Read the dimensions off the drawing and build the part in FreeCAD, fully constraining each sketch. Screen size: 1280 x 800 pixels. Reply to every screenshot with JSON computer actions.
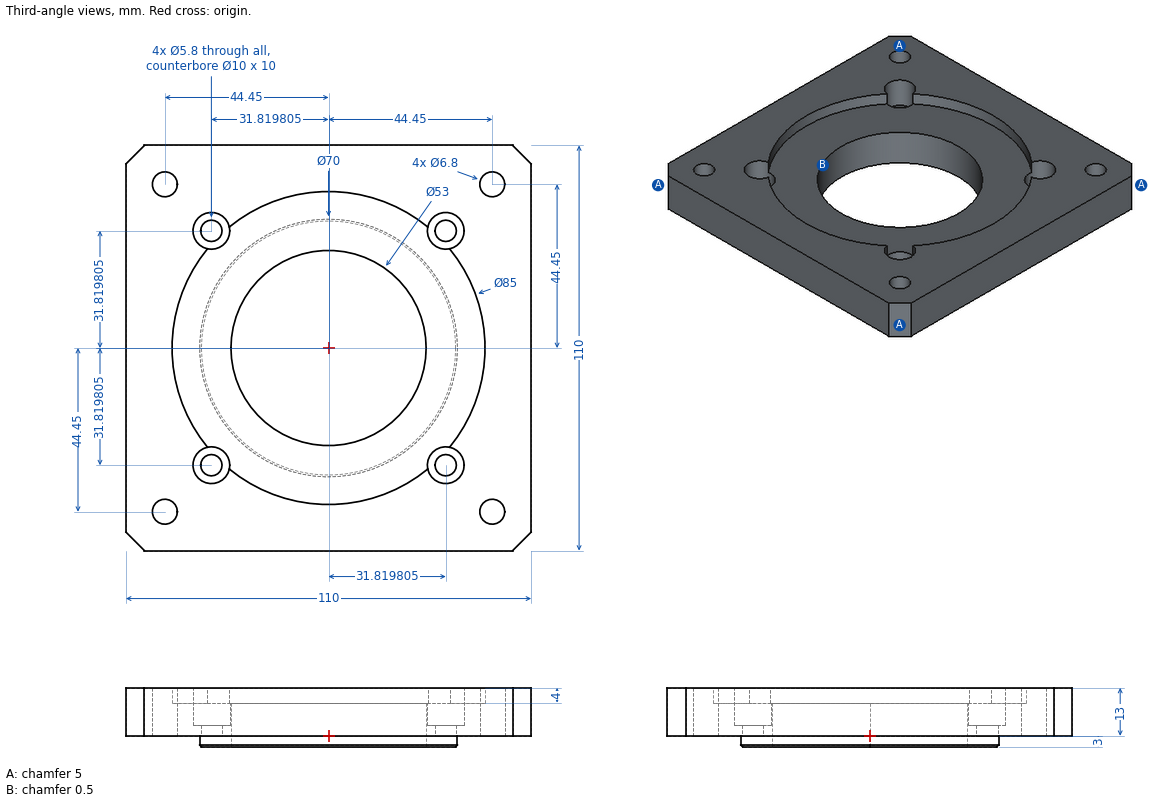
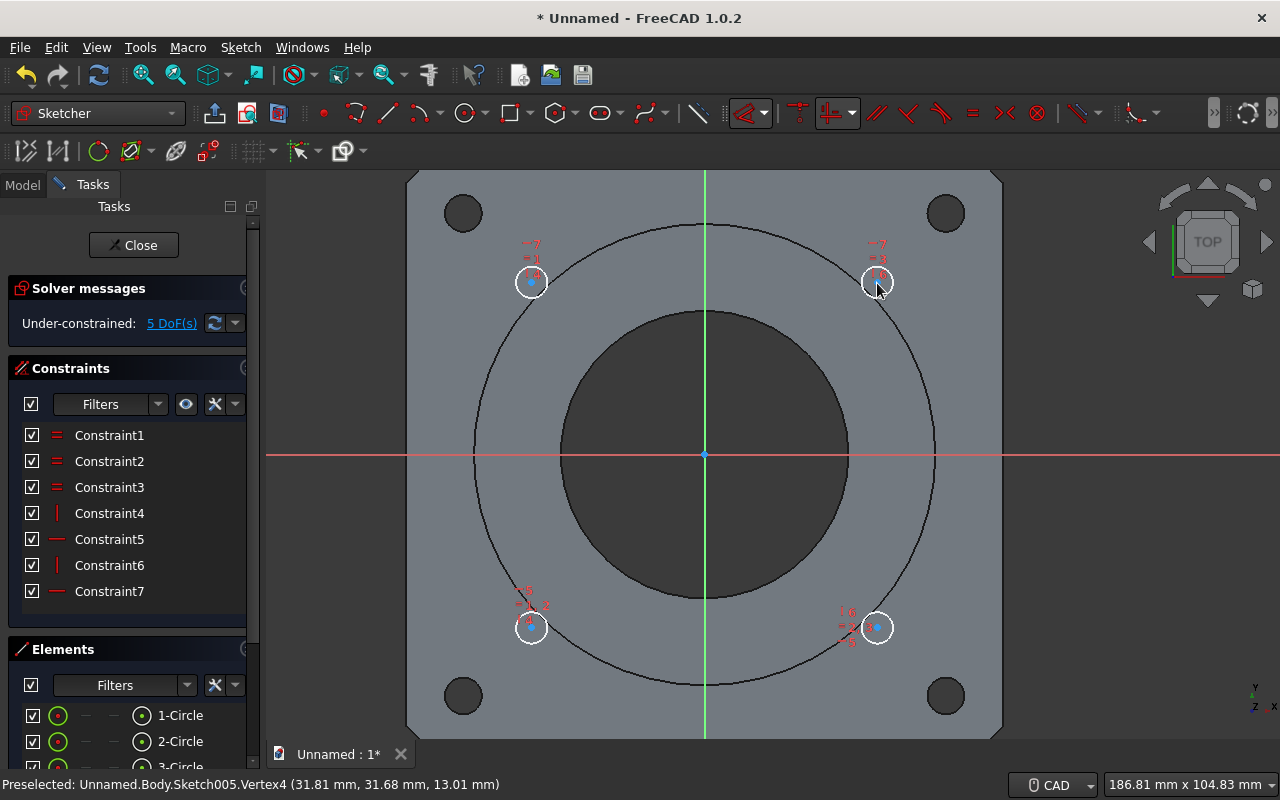
{"action": "scroll", "coordinate": [543, 271], "scroll_direction": "up", "scroll_amount": 2}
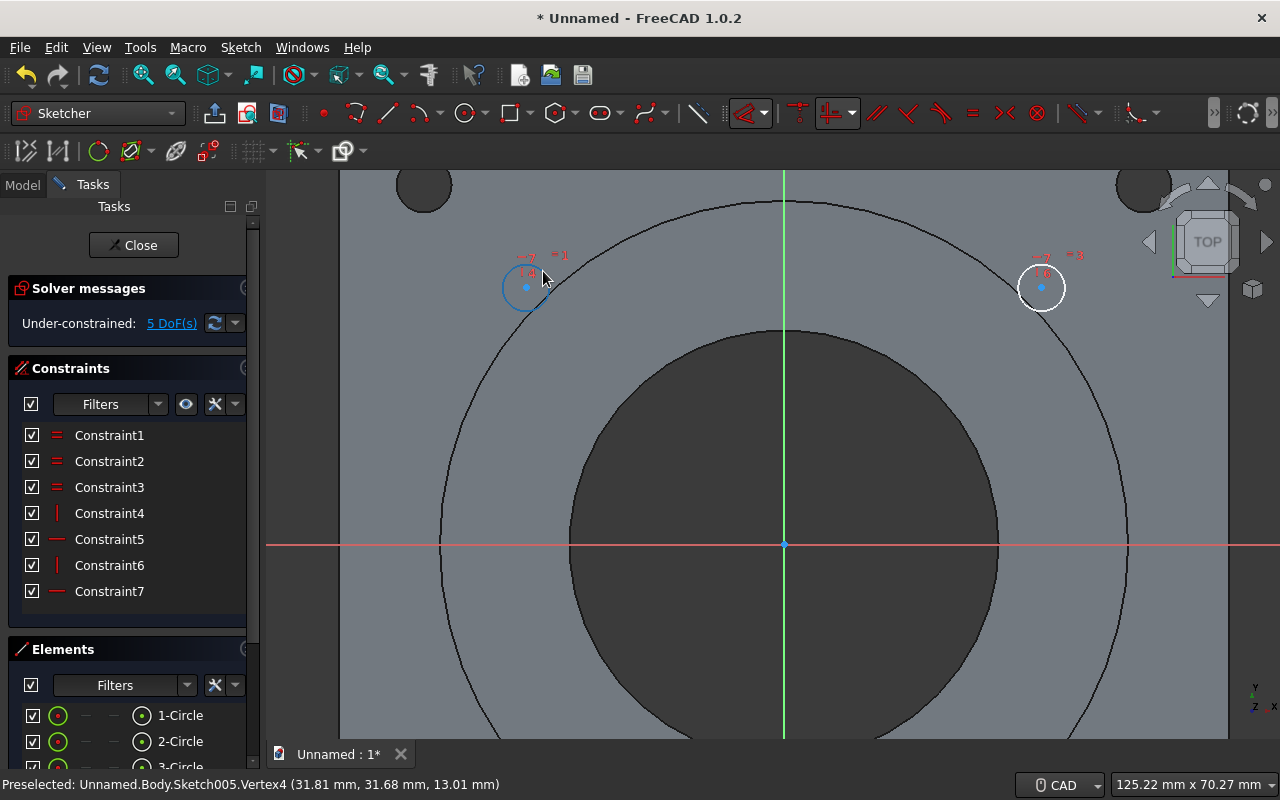
{"action": "left_click", "coordinate": [543, 271]}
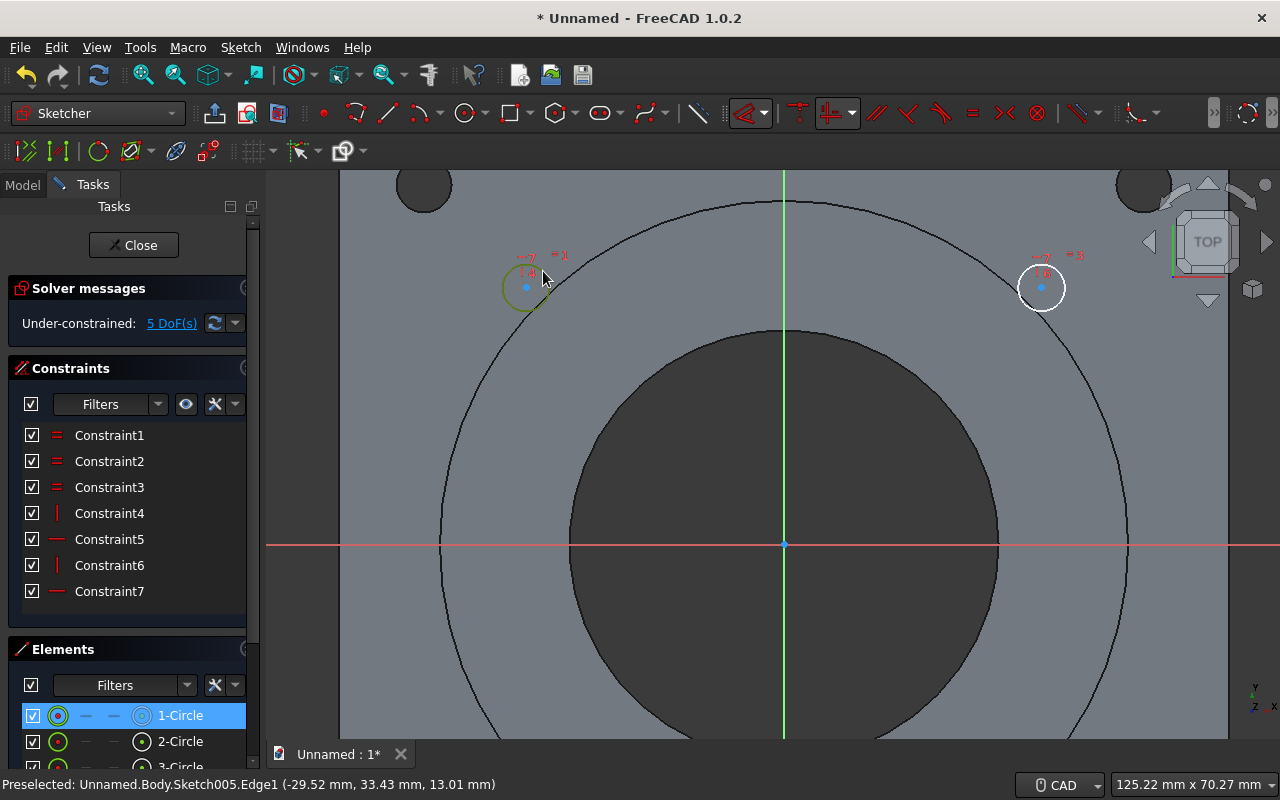
{"action": "key", "text": "k o"}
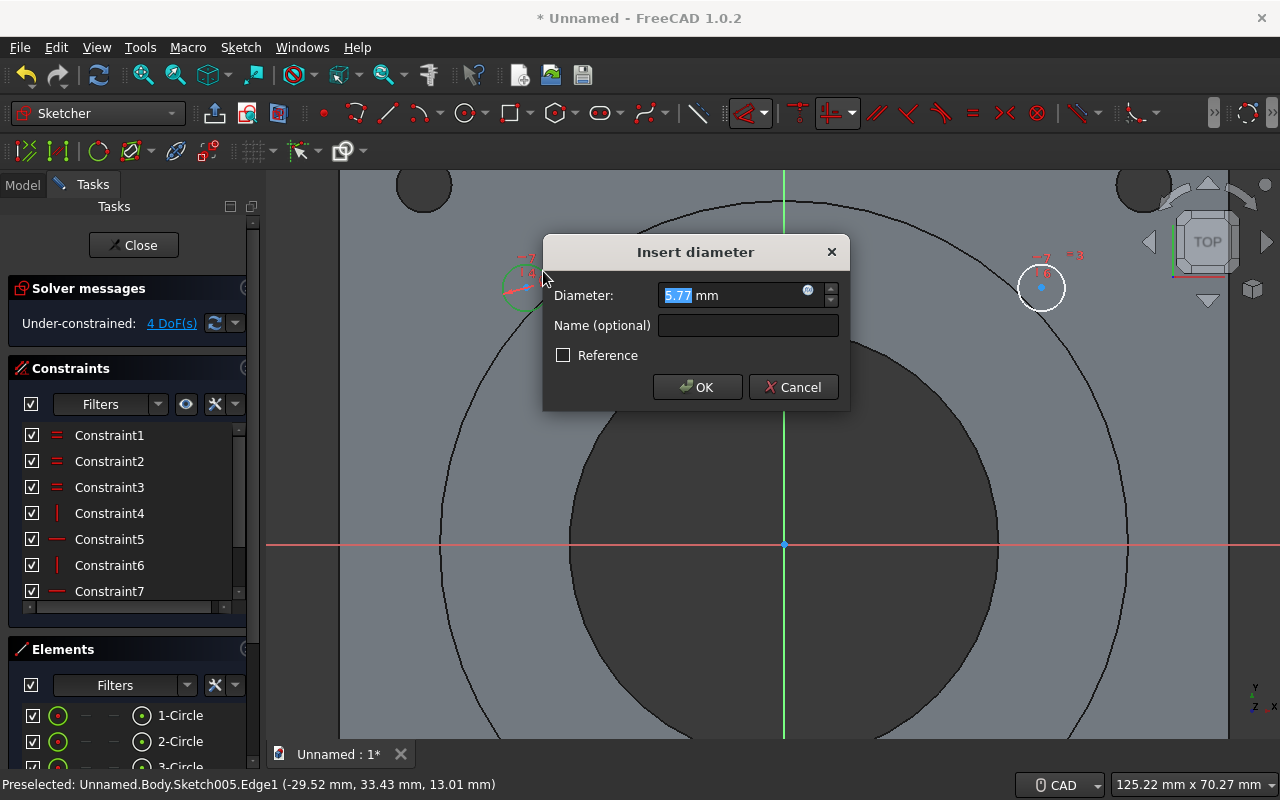
{"action": "type", "text": "5.8"}
{"action": "key", "text": "Return"}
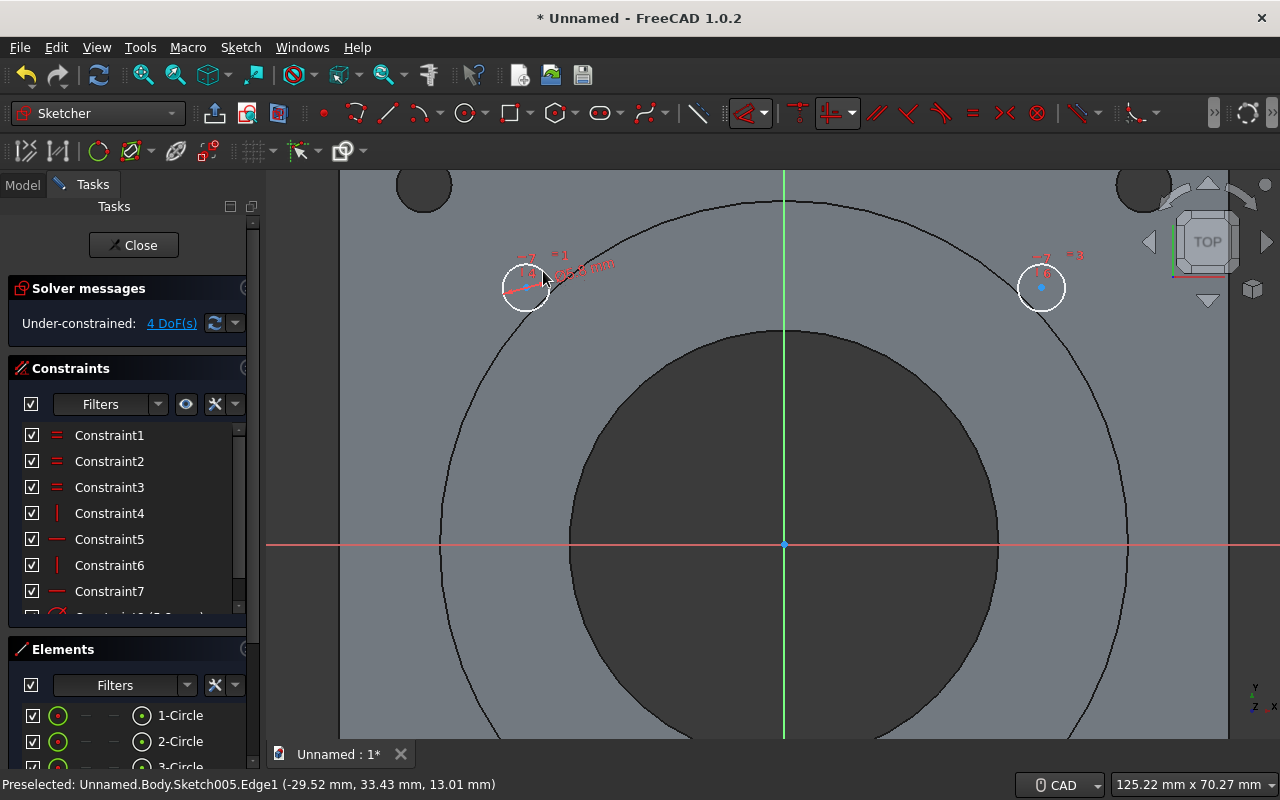
{"action": "left_click", "coordinate": [526, 288]}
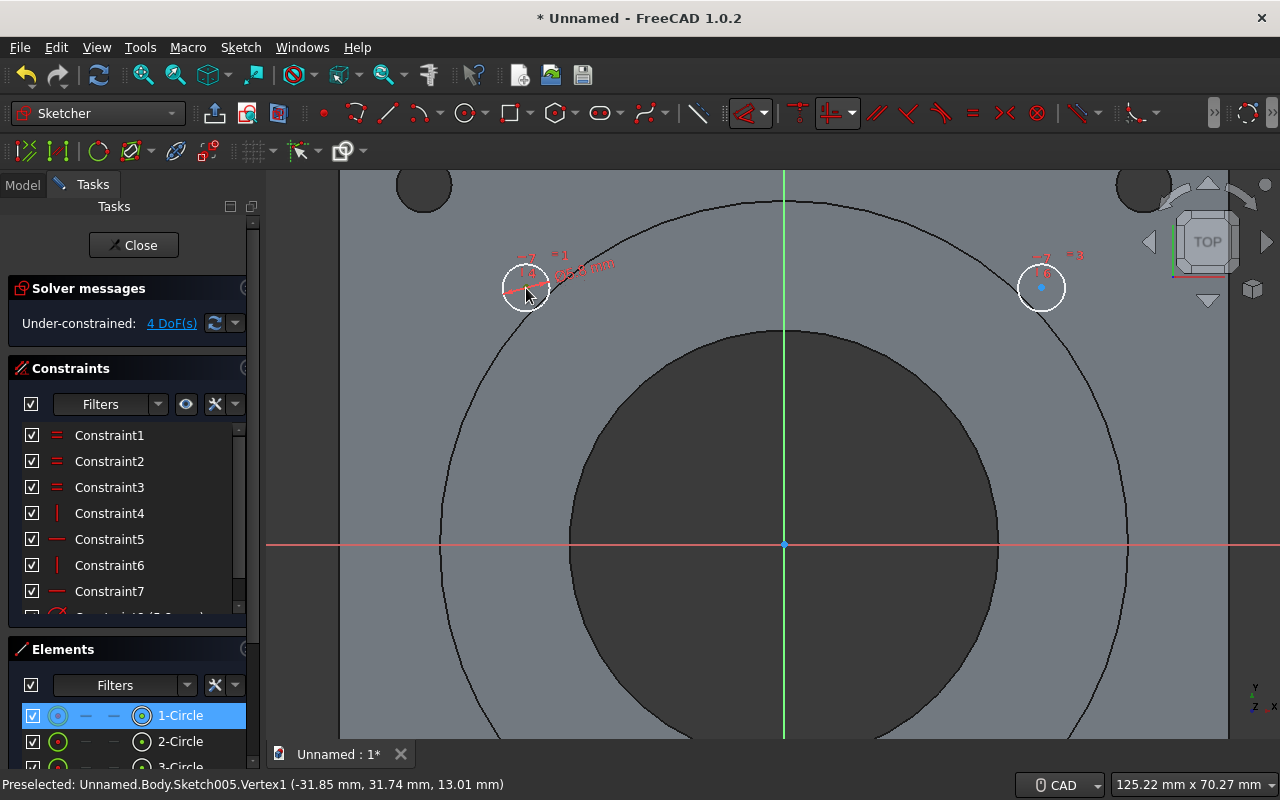
{"action": "key", "text": "l"}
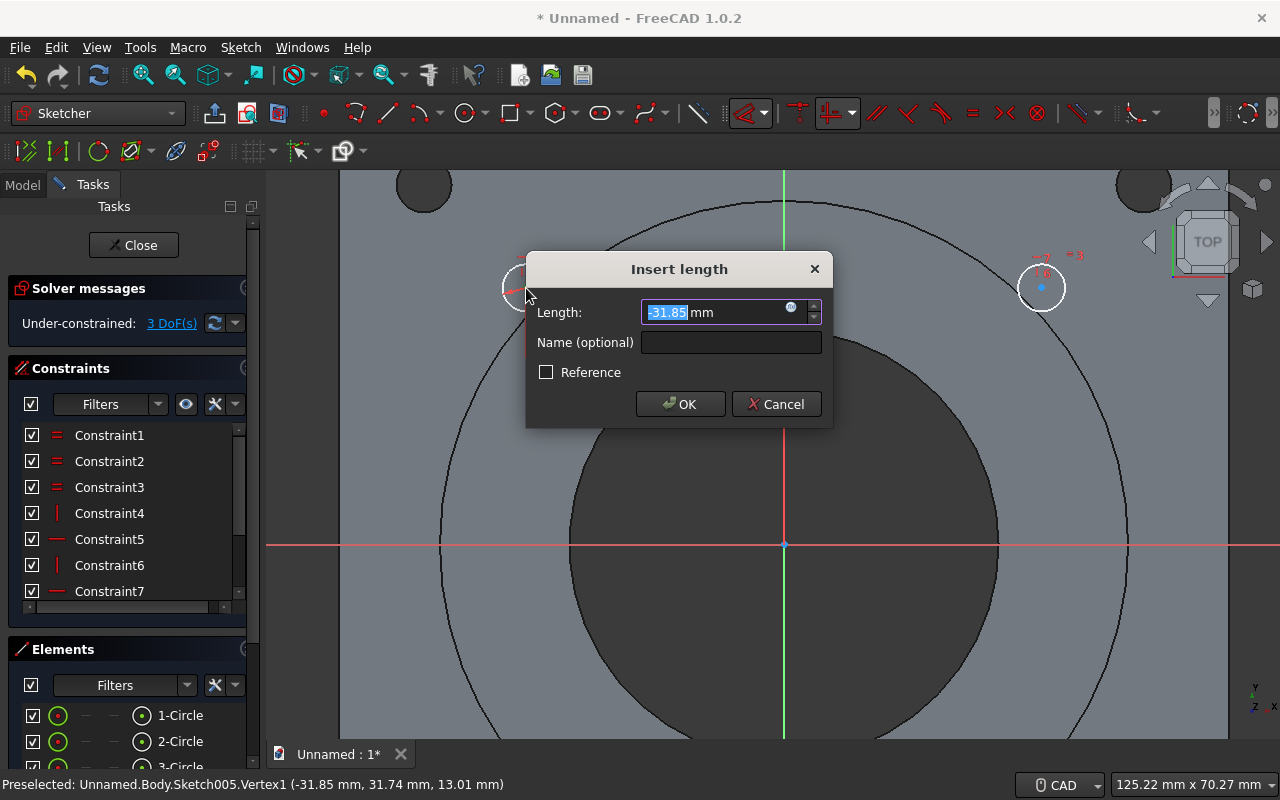
{"action": "type", "text": "-31.819805"}
{"action": "key", "text": "Return"}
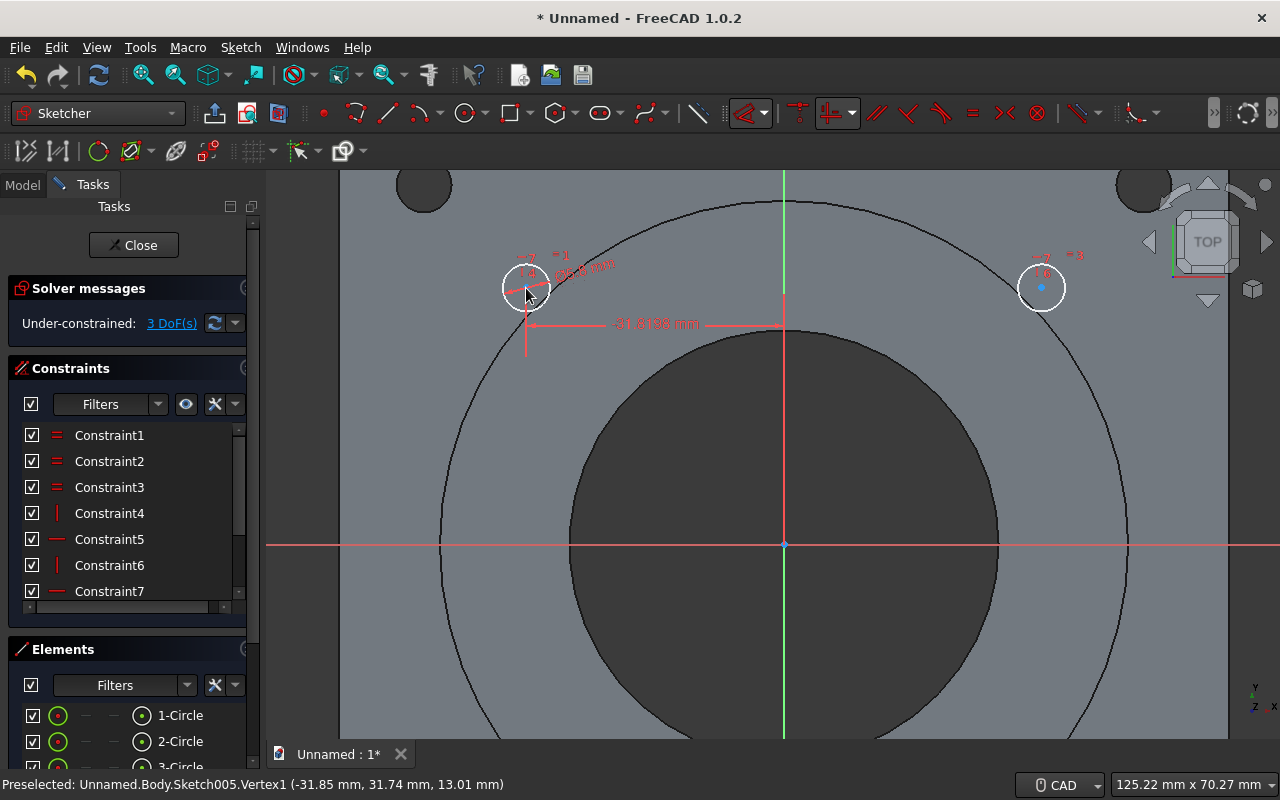
{"action": "left_click", "coordinate": [526, 288]}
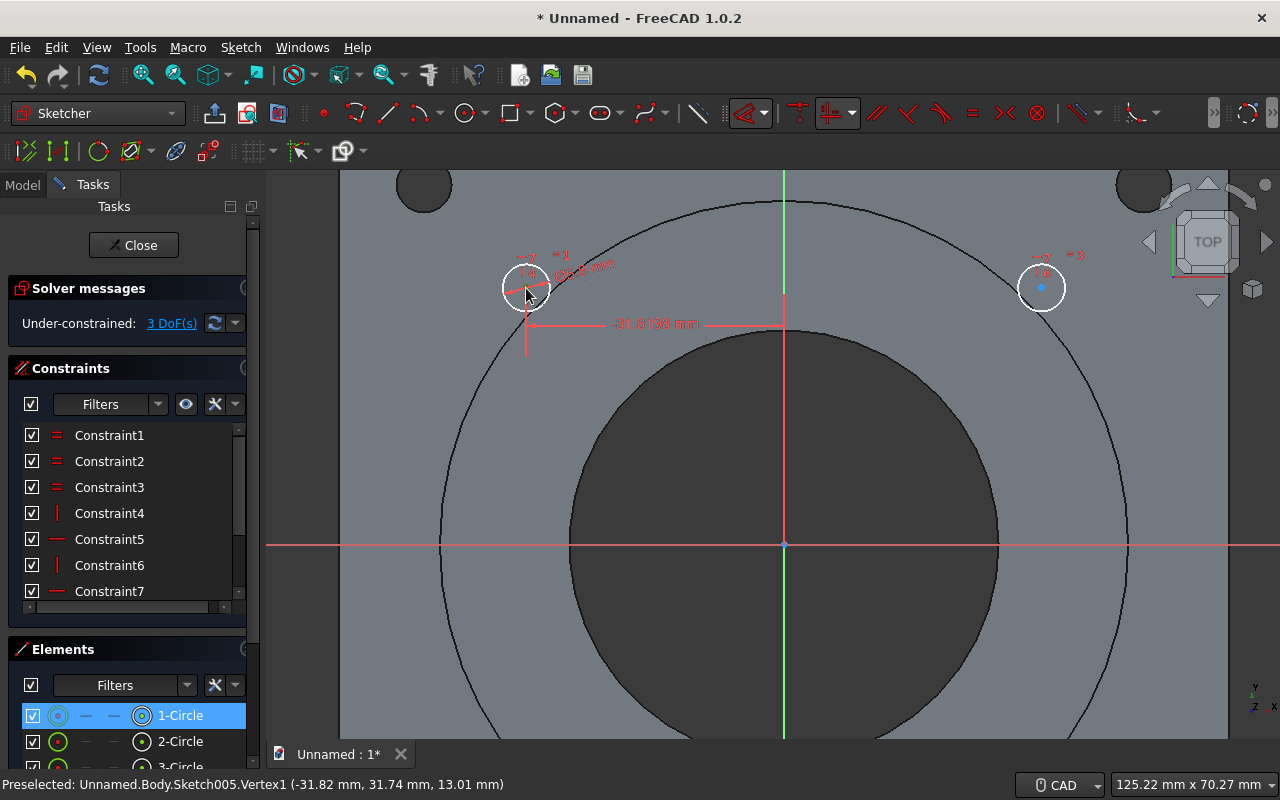
{"action": "left_click", "coordinate": [766, 114]}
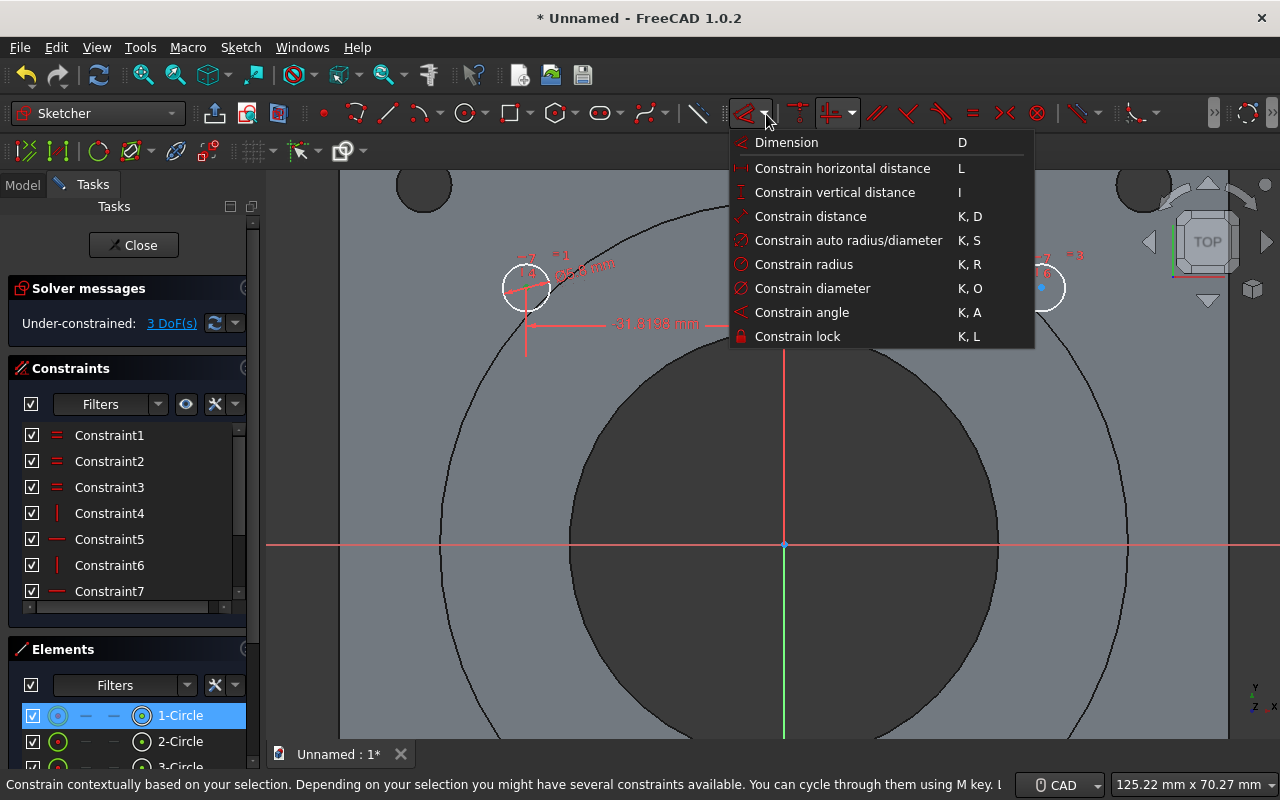
{"action": "left_click", "coordinate": [882, 192]}